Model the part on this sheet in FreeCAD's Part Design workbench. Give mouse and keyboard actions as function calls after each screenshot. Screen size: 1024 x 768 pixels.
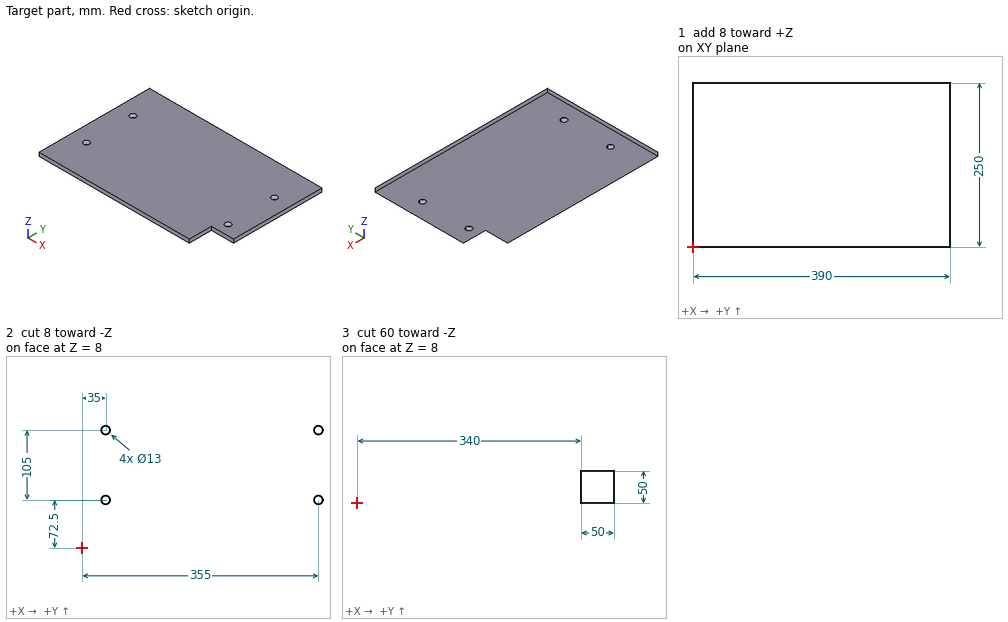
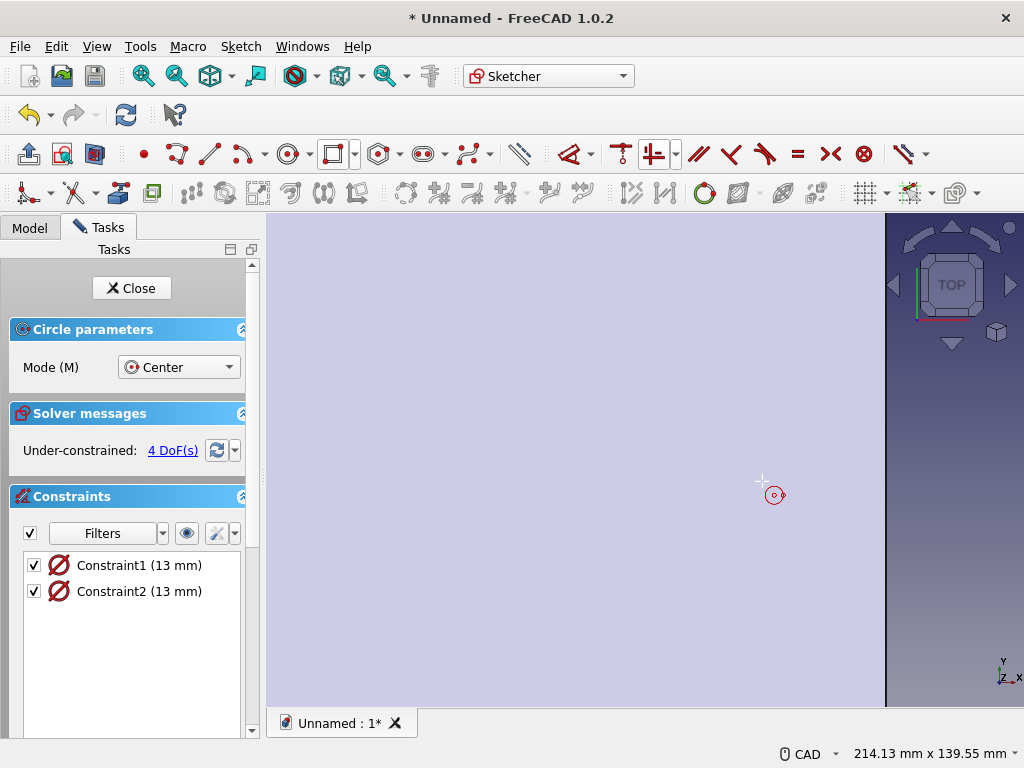
click(762, 480)
move(778, 463)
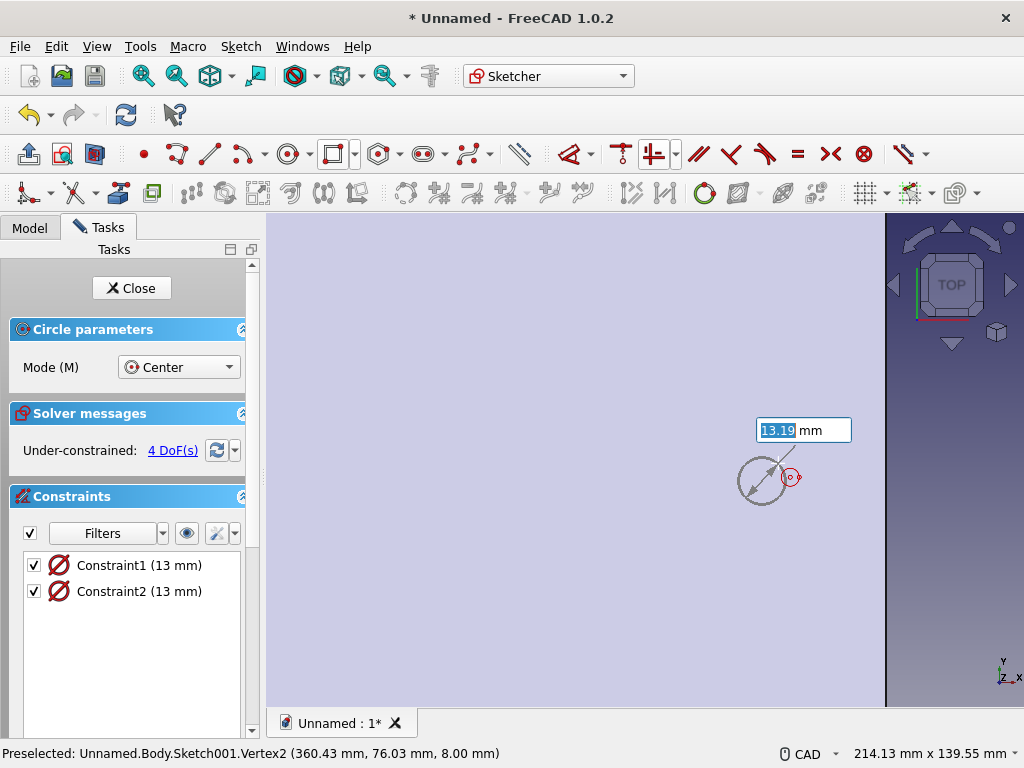
text(13)
key(Return)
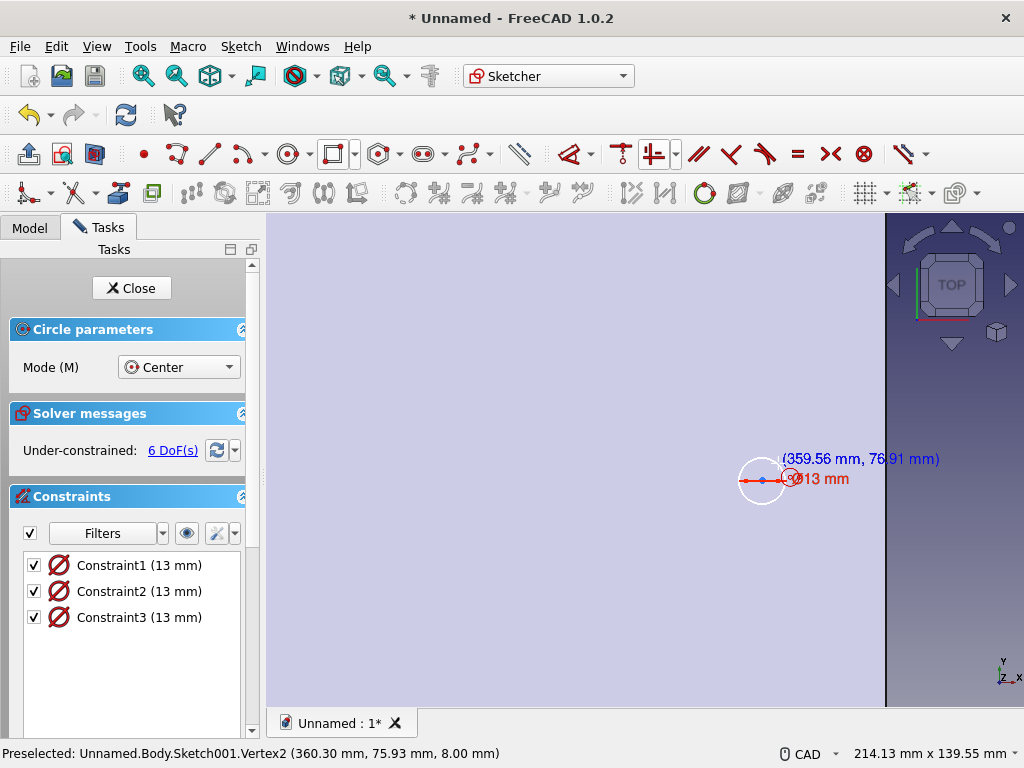
scroll(762, 481, down, 6)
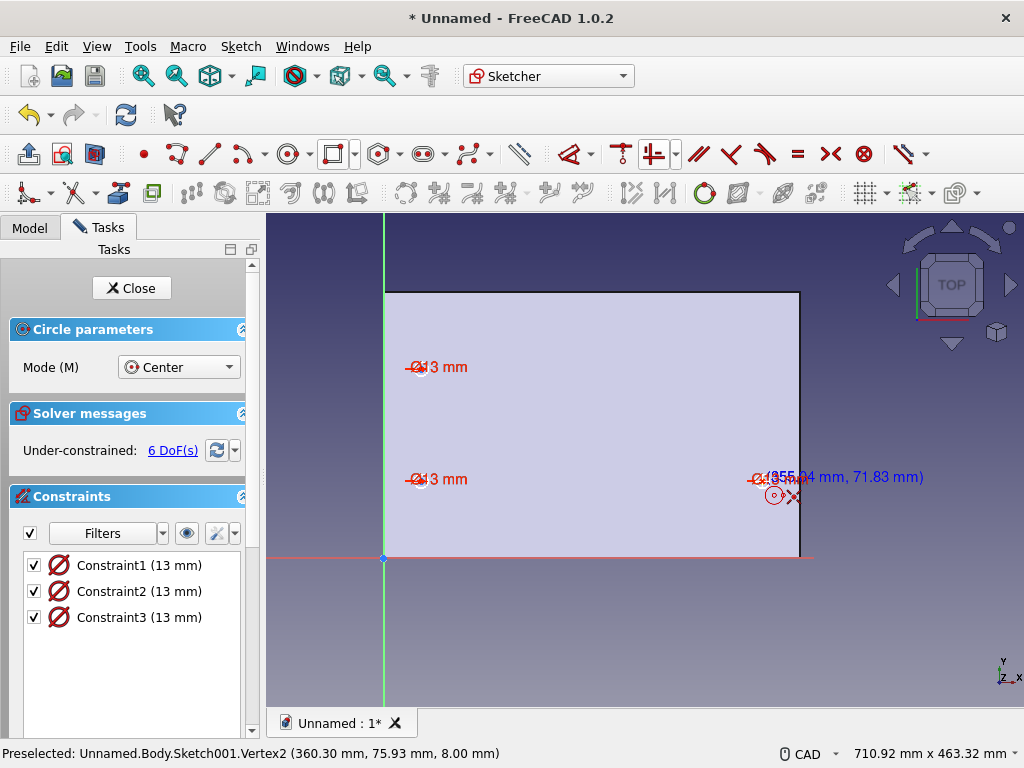
scroll(762, 369, up, 6)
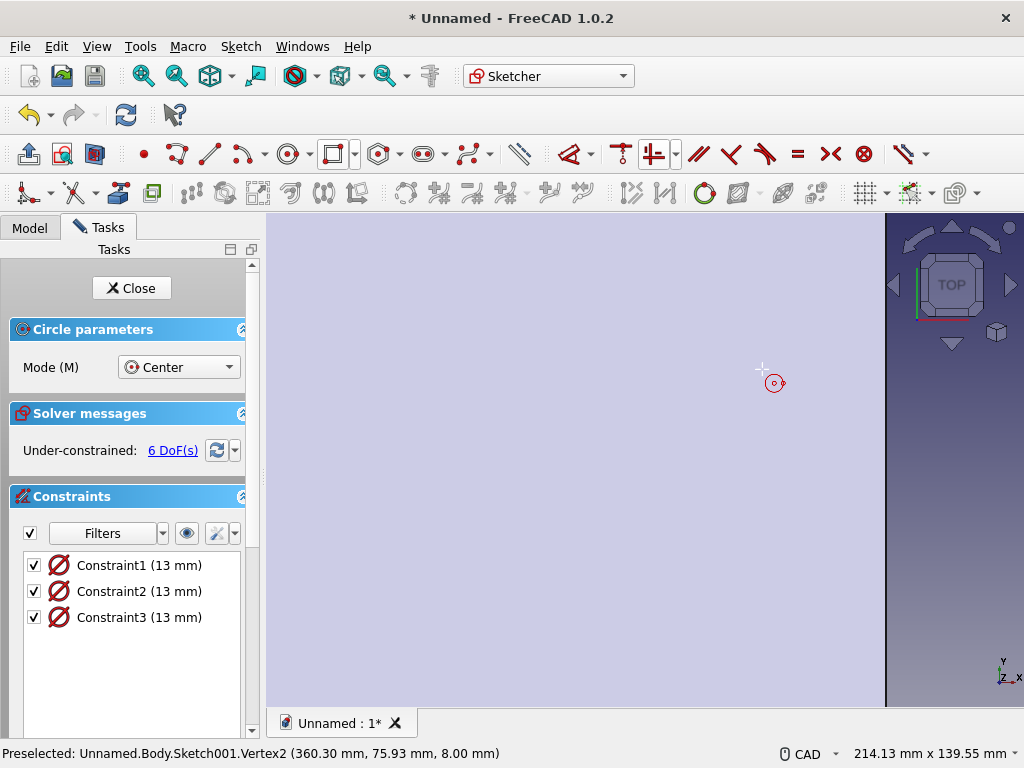
click(762, 368)
move(778, 352)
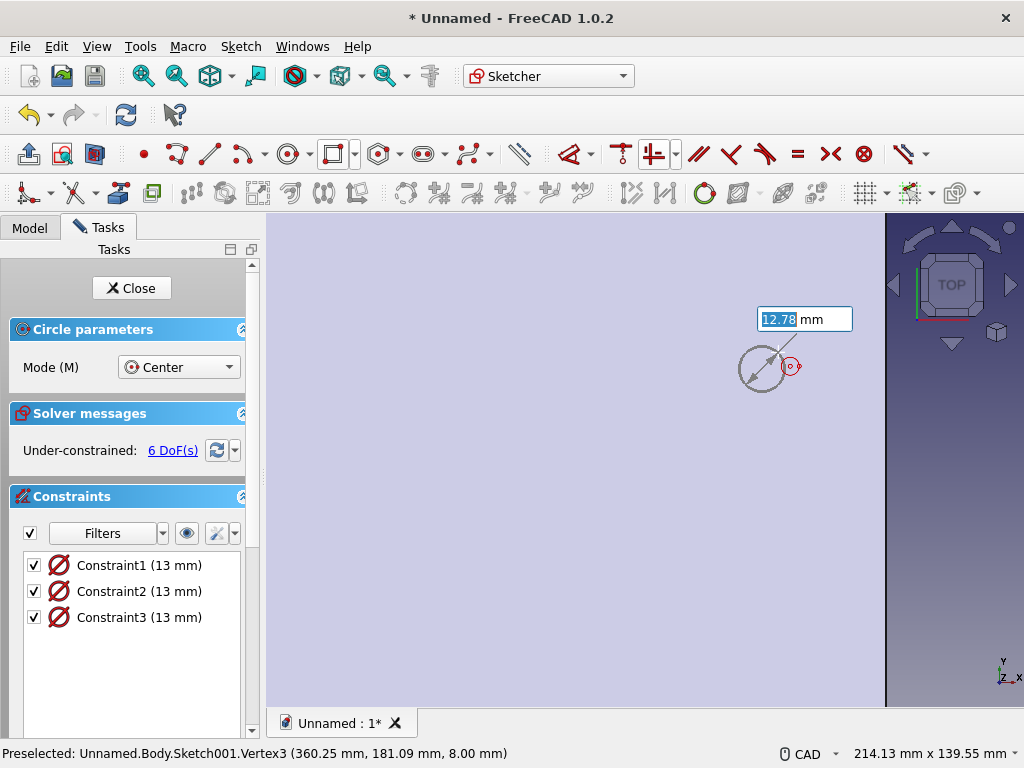
text(13)
key(Return)
key(Escape)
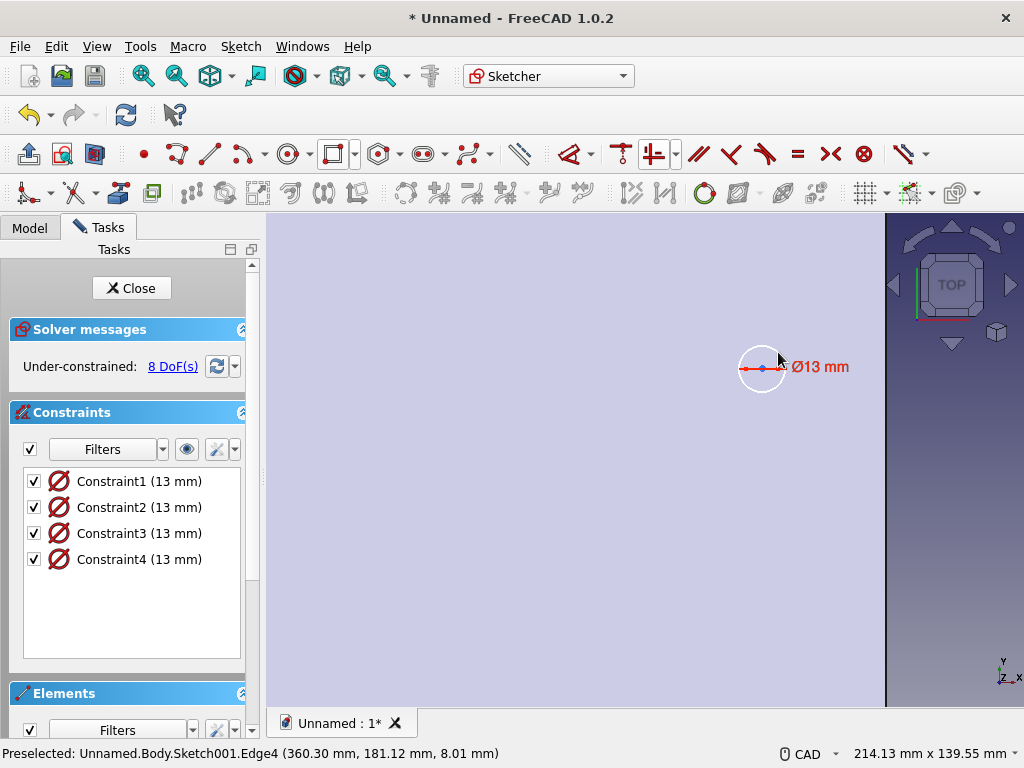
scroll(762, 369, down, 6)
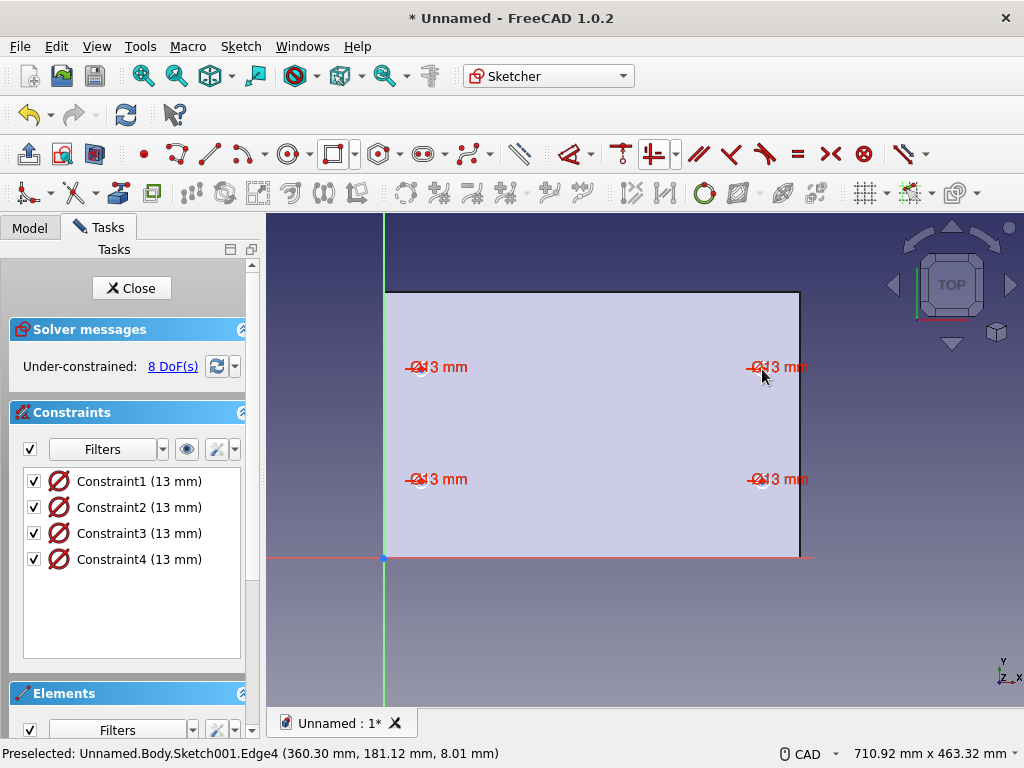
click(421, 369)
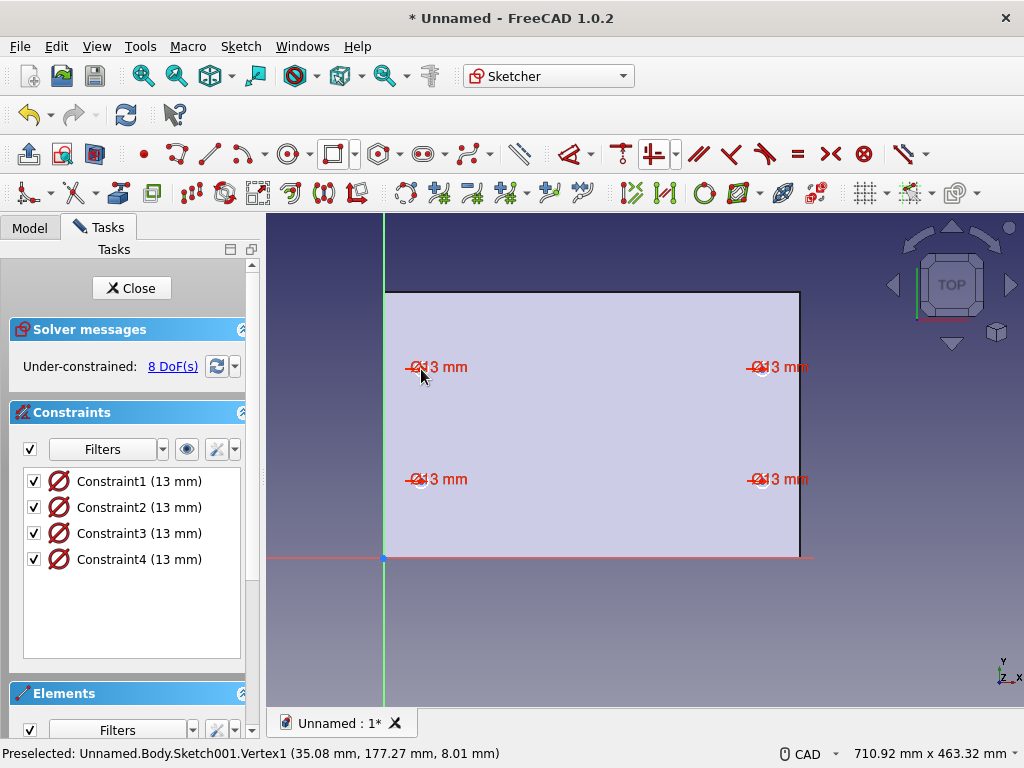
click(421, 481)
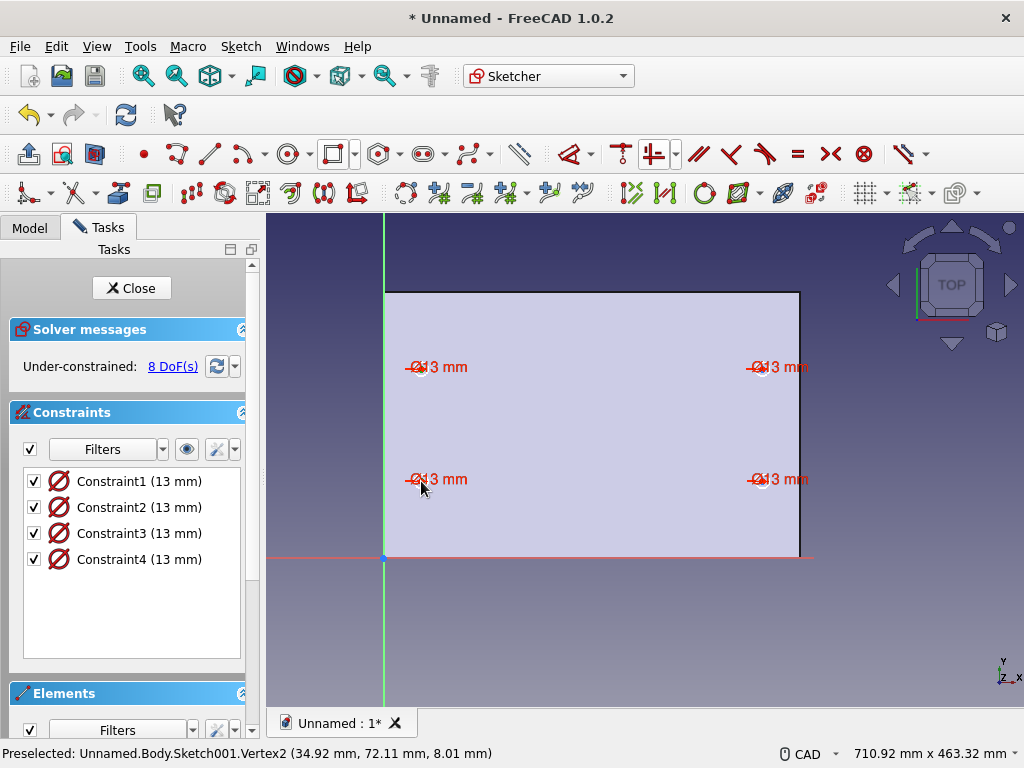
key(v)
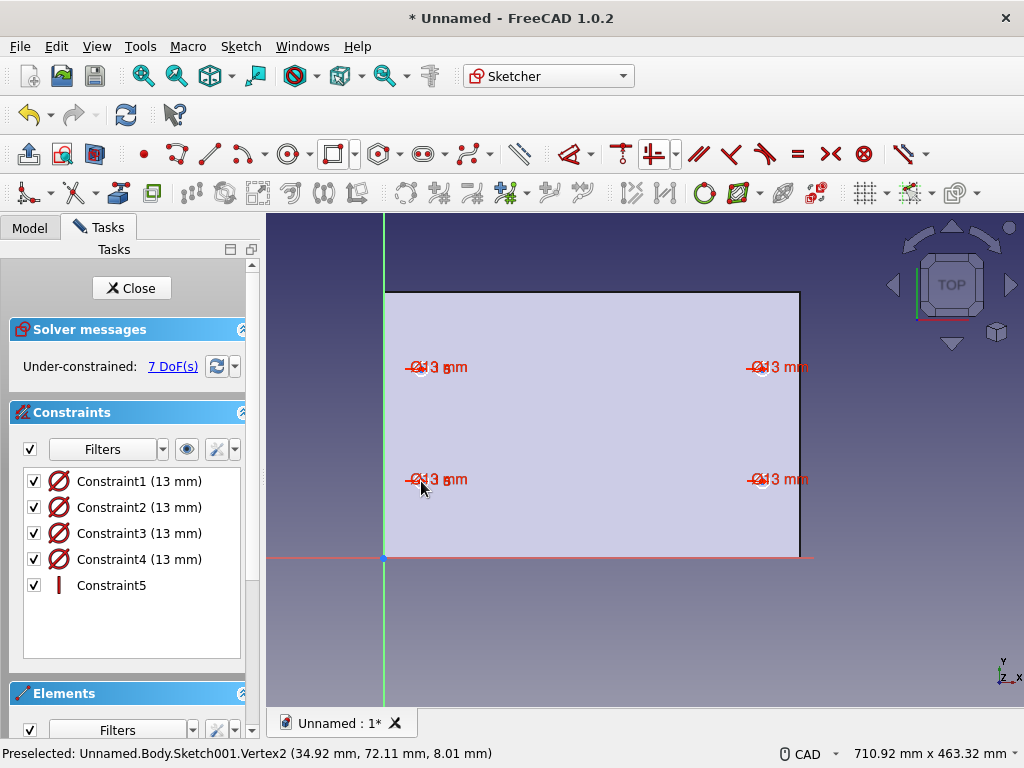
click(421, 481)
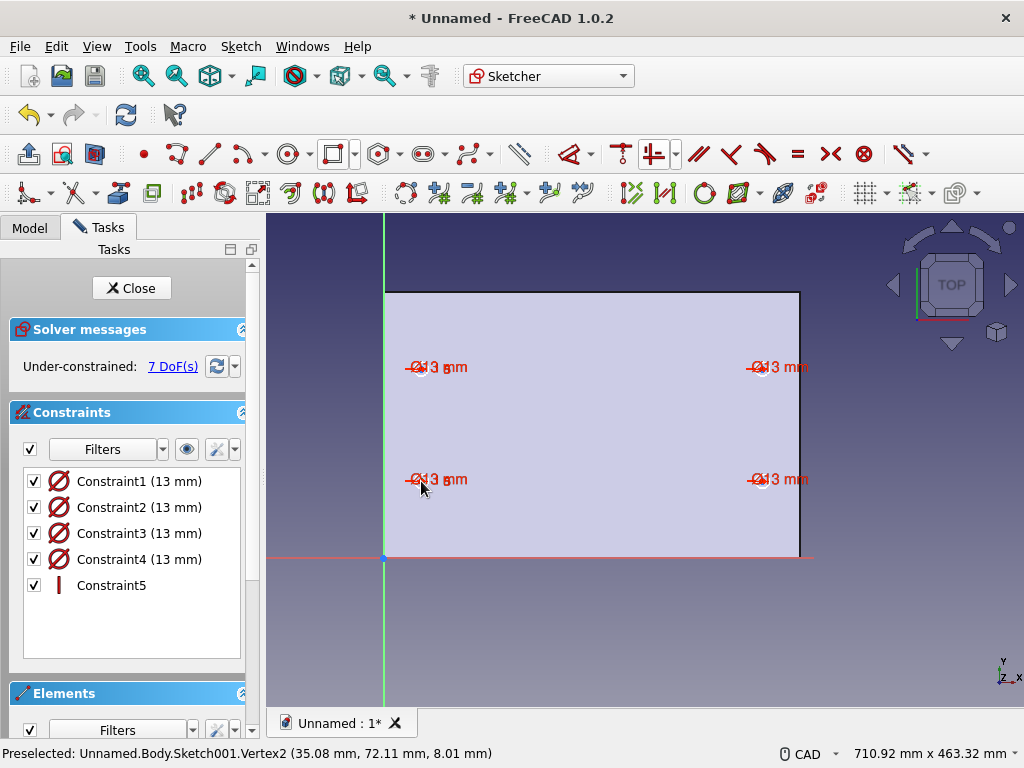
click(762, 481)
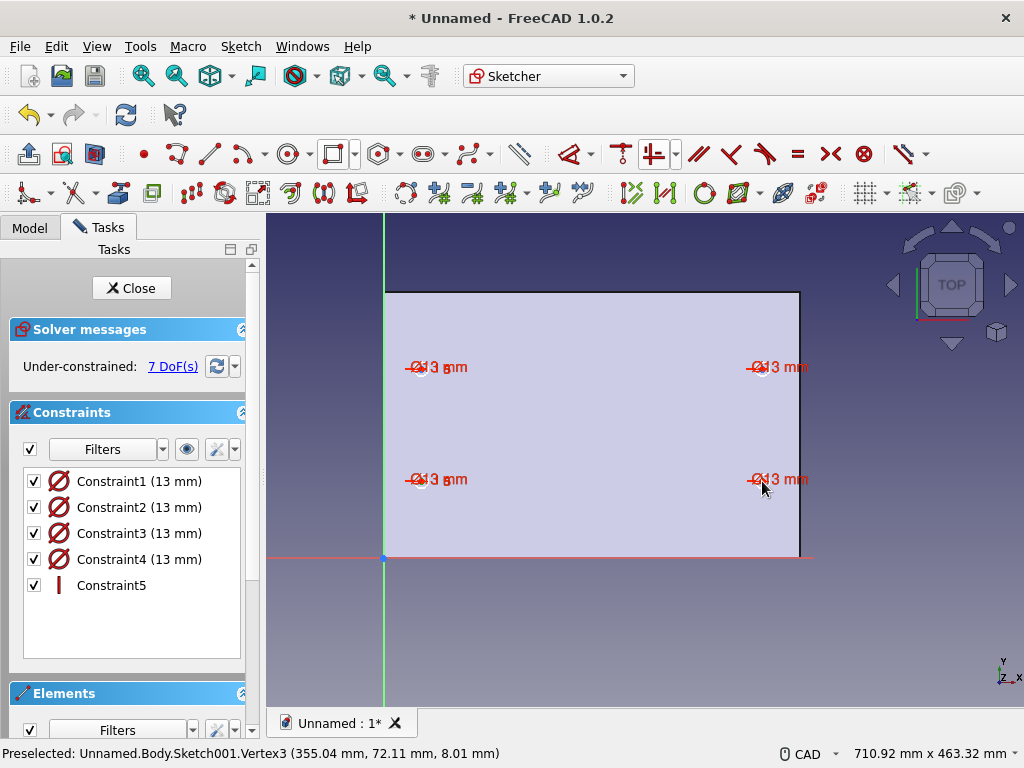
key(h)